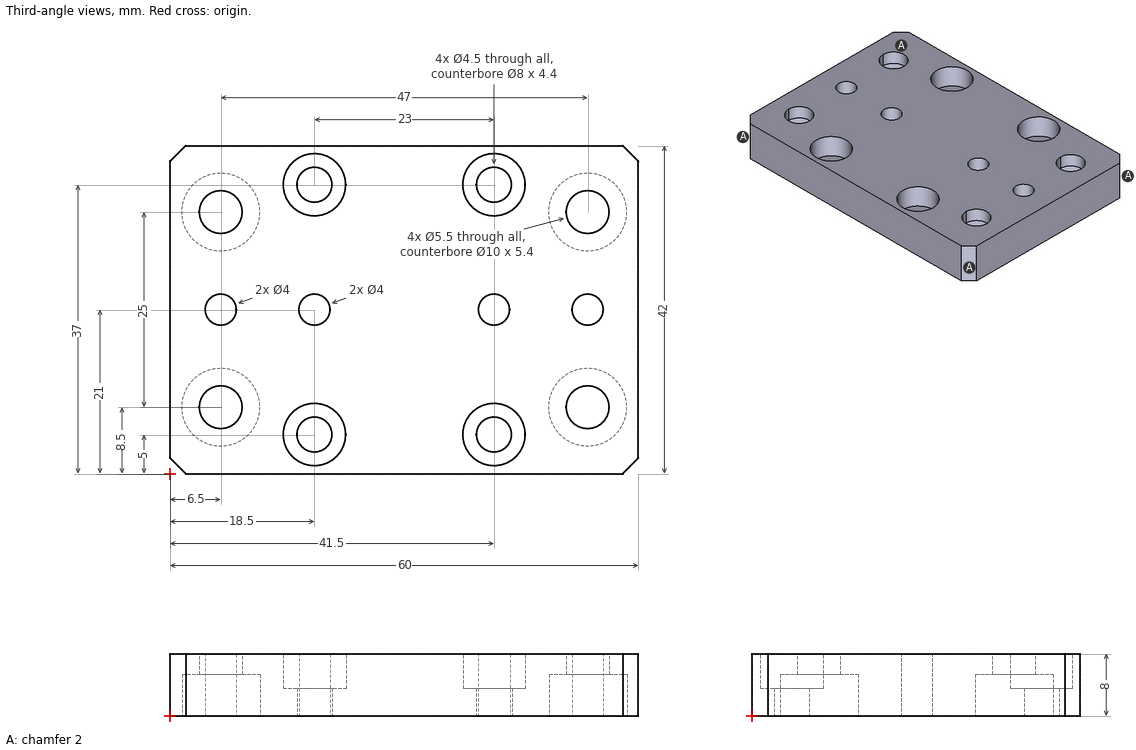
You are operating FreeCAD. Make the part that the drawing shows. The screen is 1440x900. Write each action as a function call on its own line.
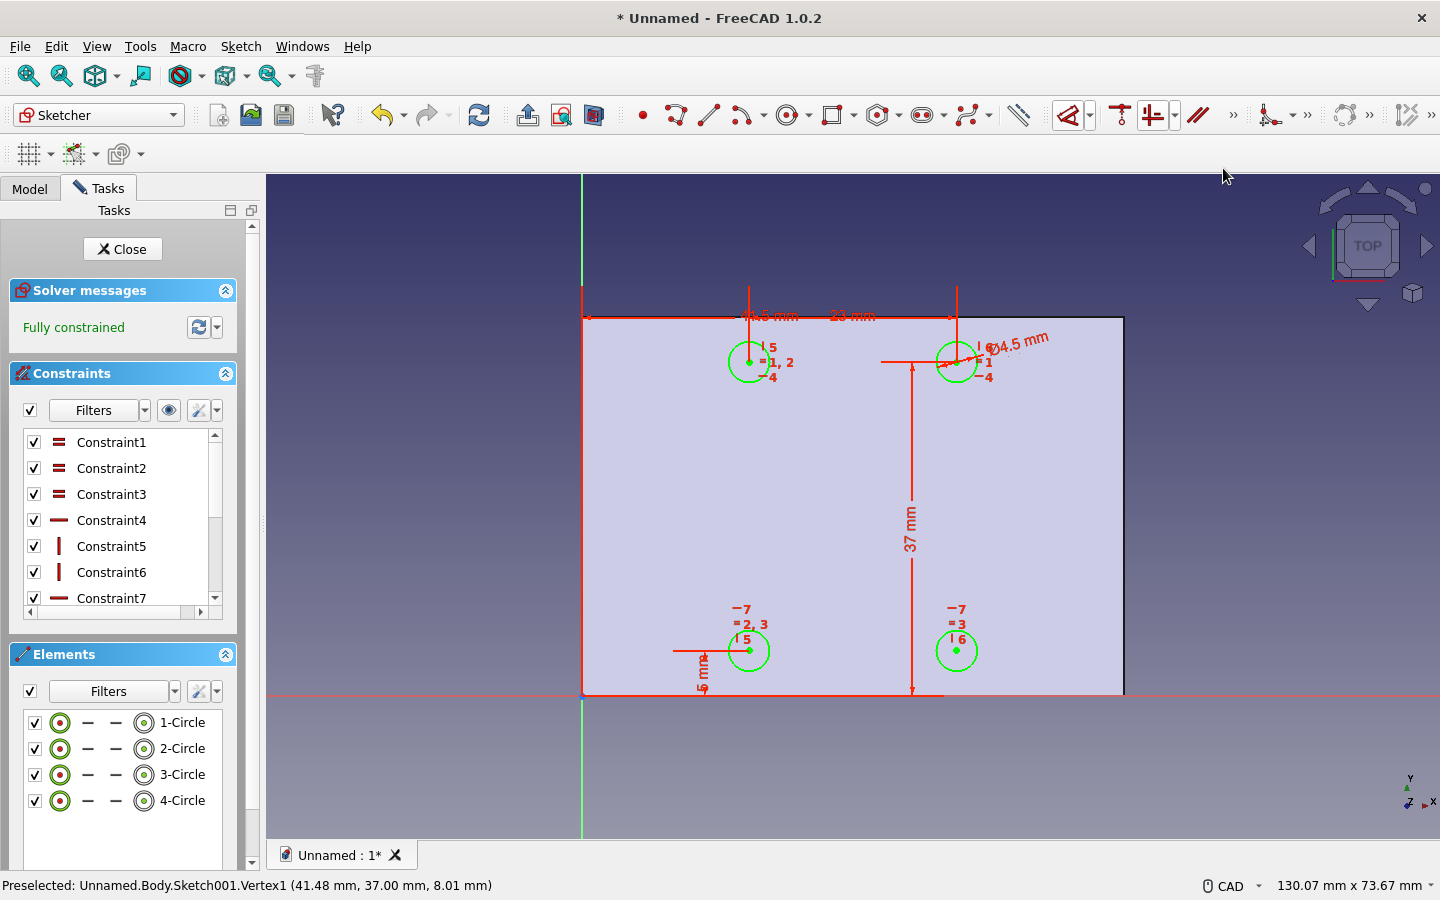
click(123, 249)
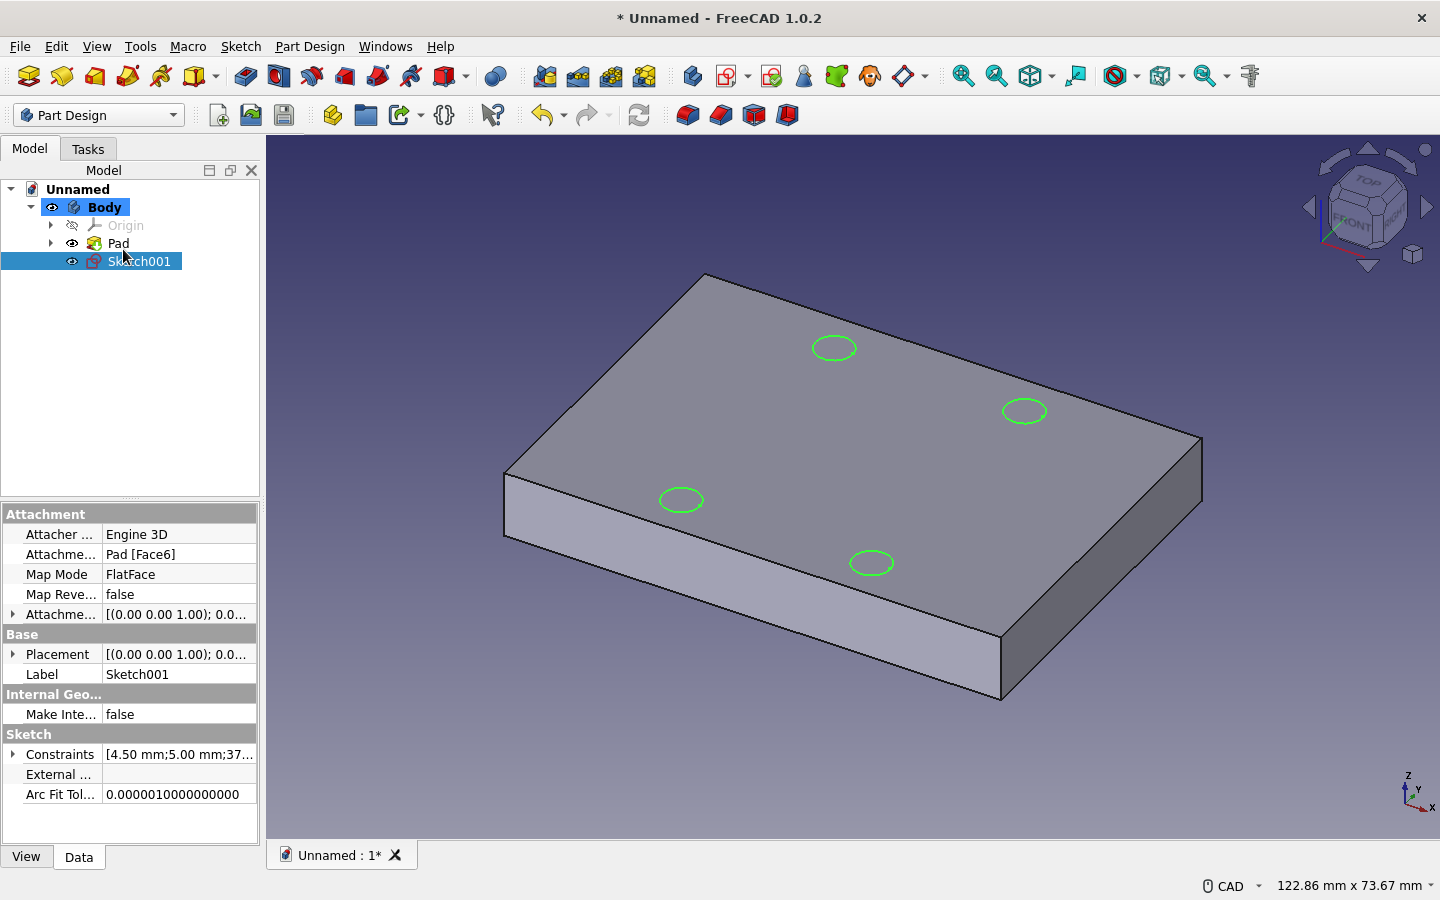
click(279, 76)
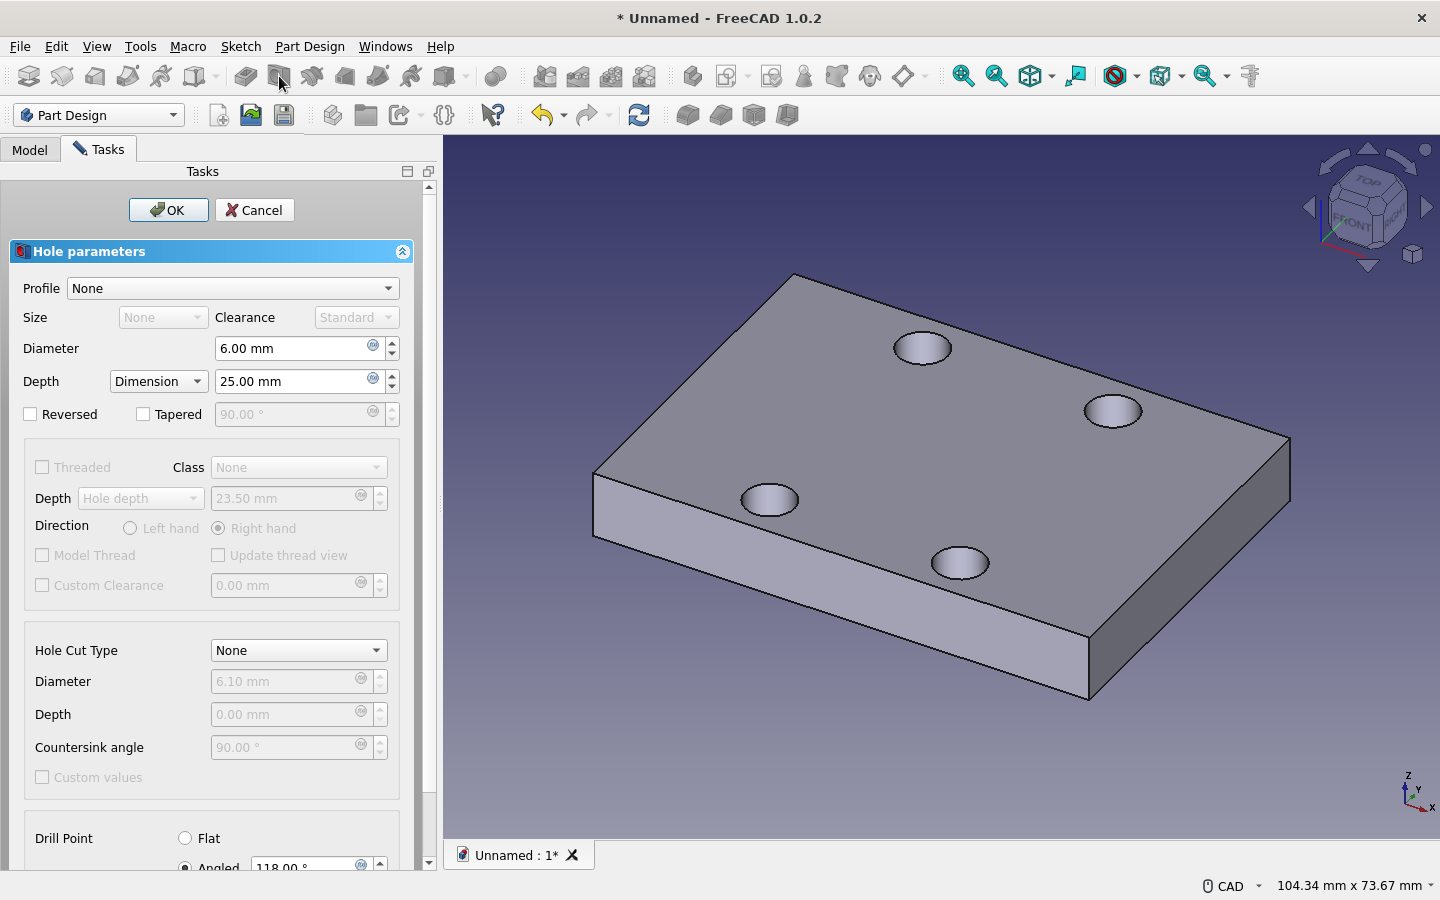
triple_click(300, 348)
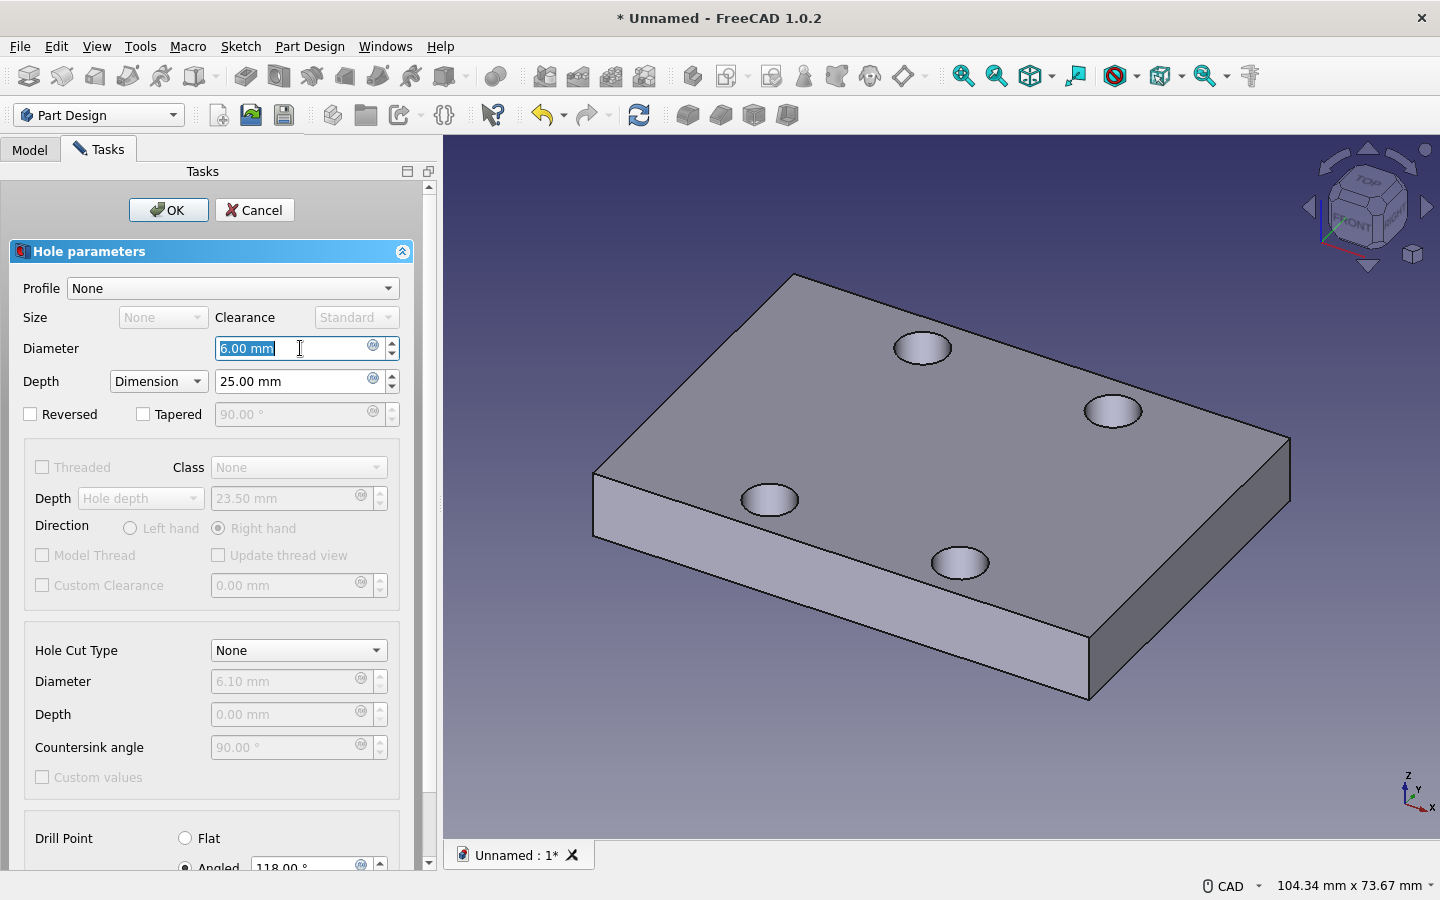
text(4.5)
key(Tab)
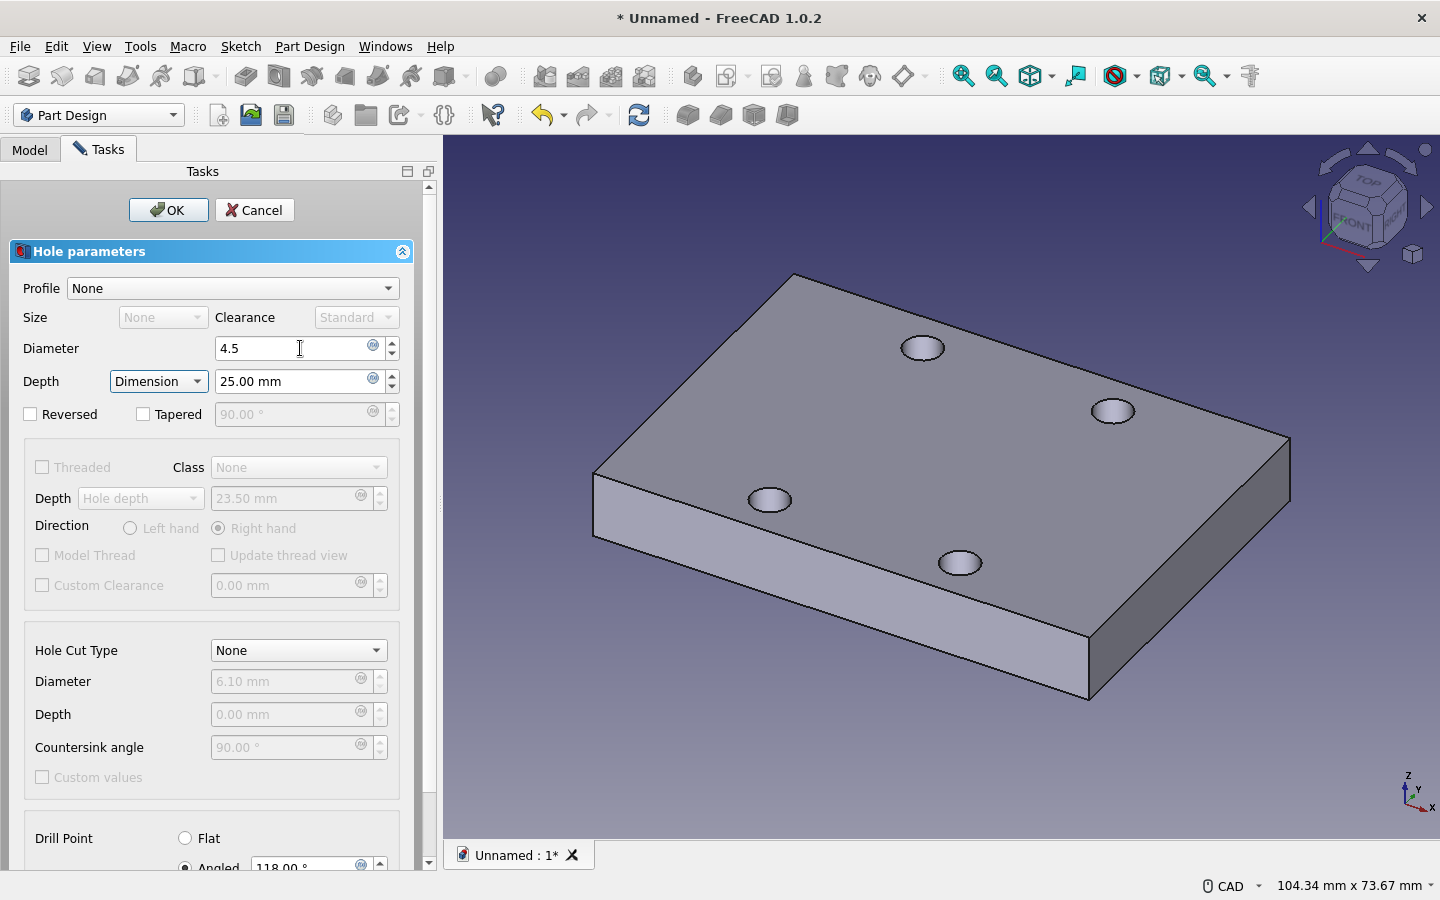
click(160, 382)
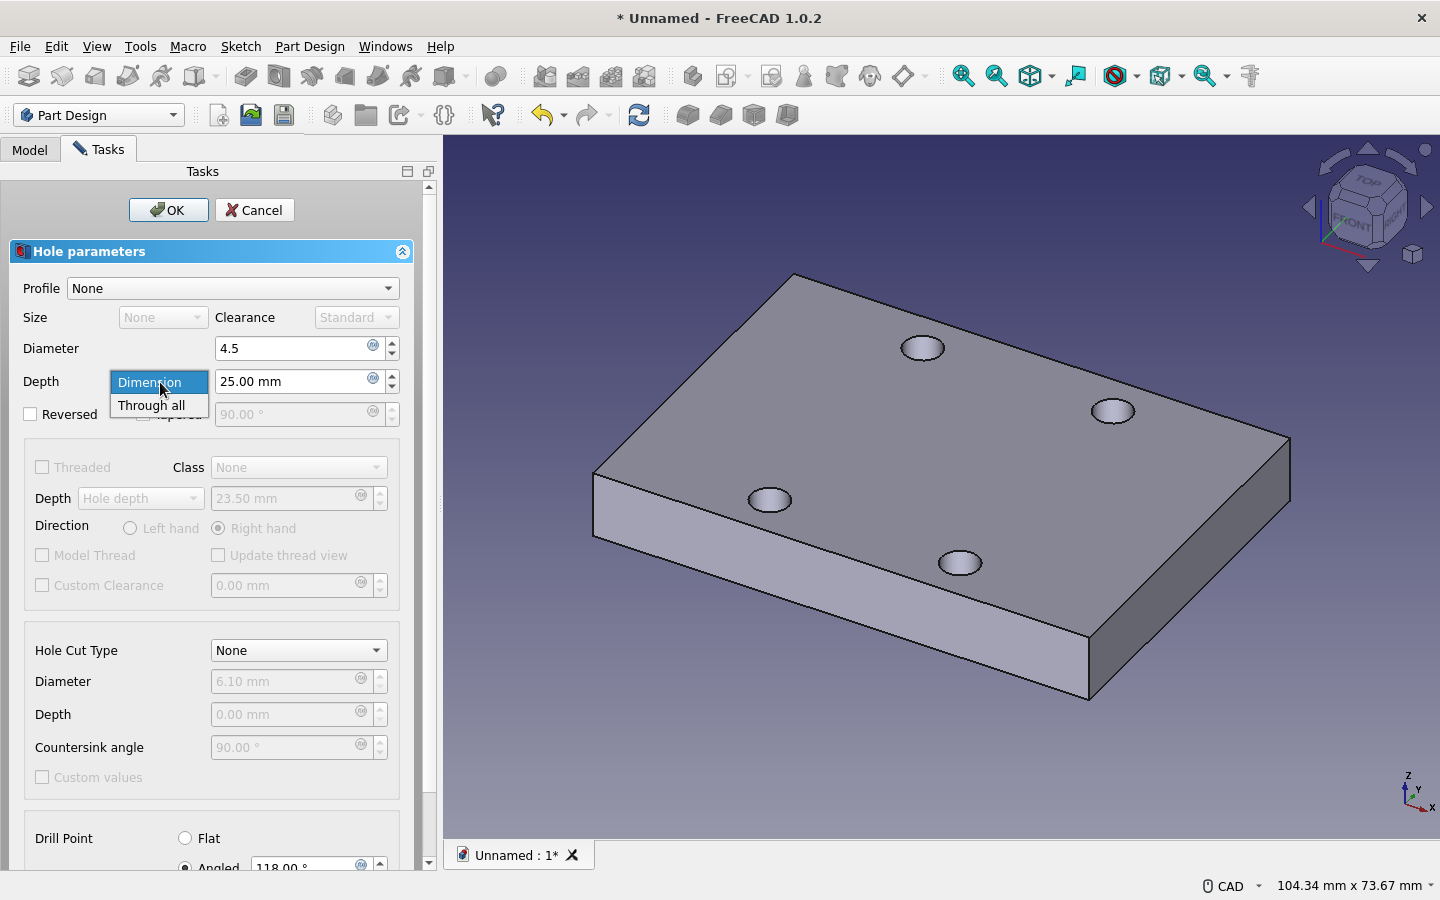
click(158, 406)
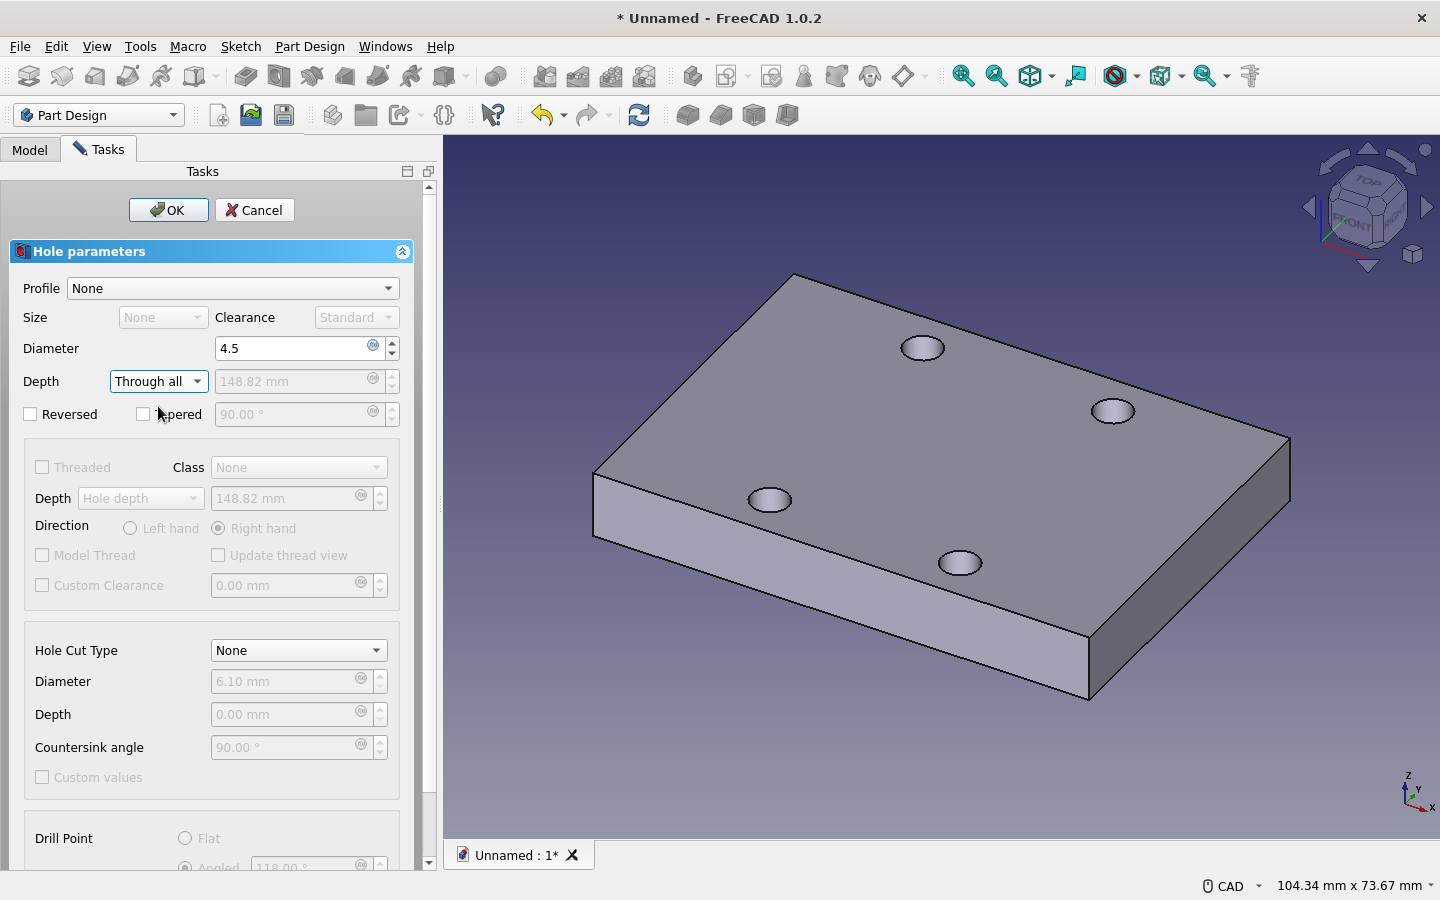
click(300, 650)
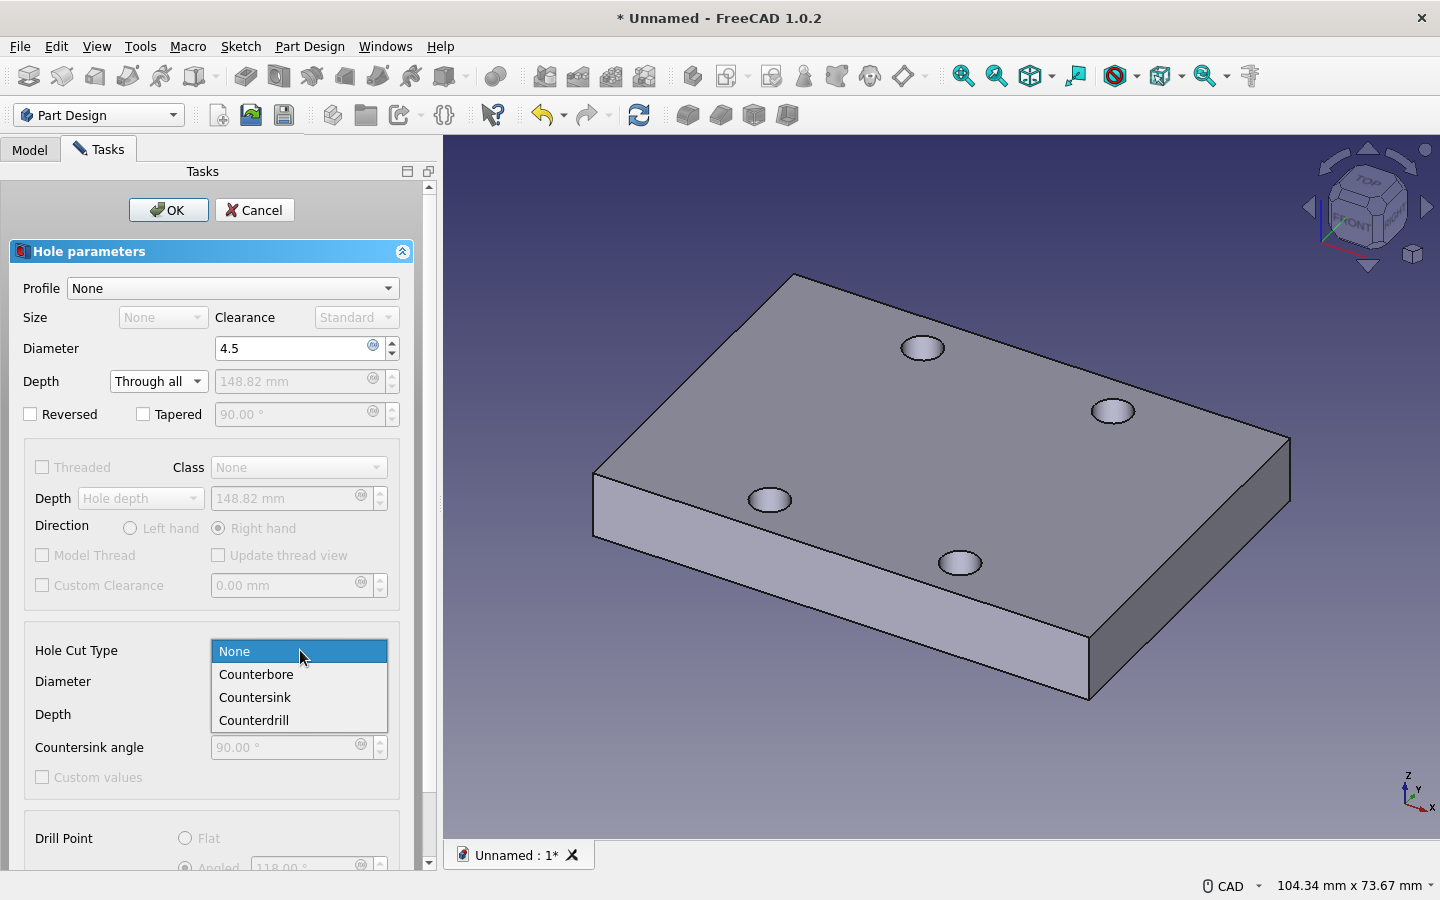
click(298, 674)